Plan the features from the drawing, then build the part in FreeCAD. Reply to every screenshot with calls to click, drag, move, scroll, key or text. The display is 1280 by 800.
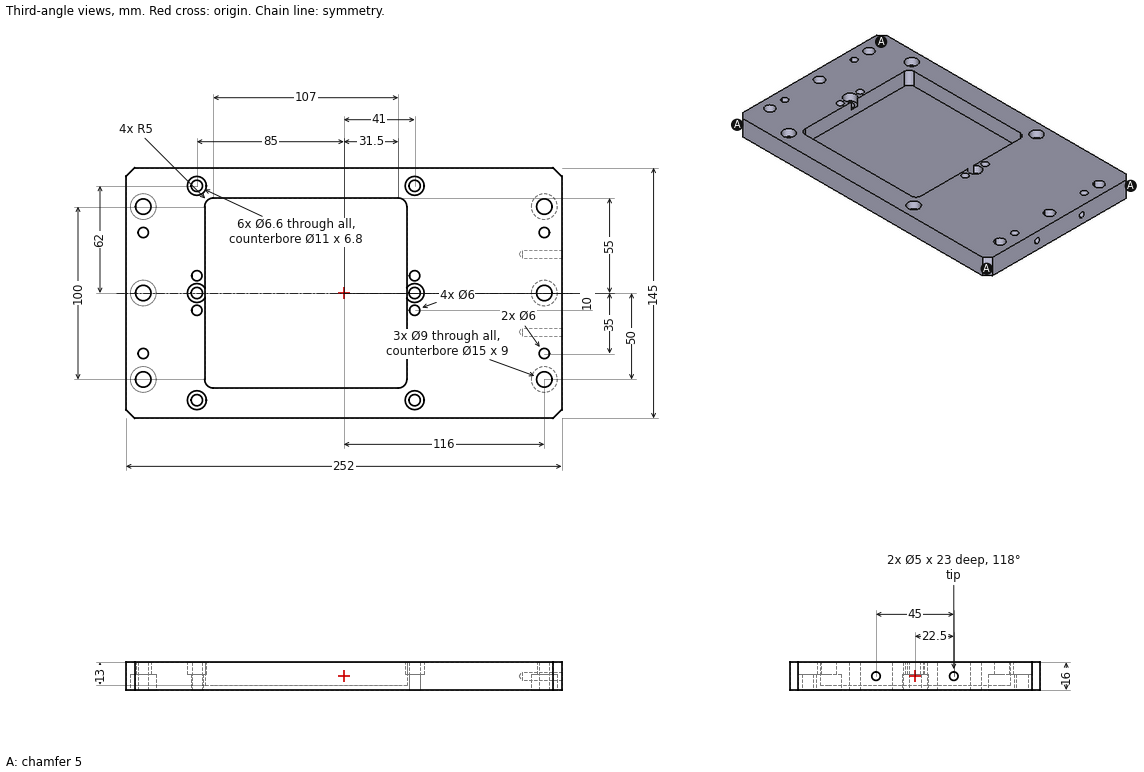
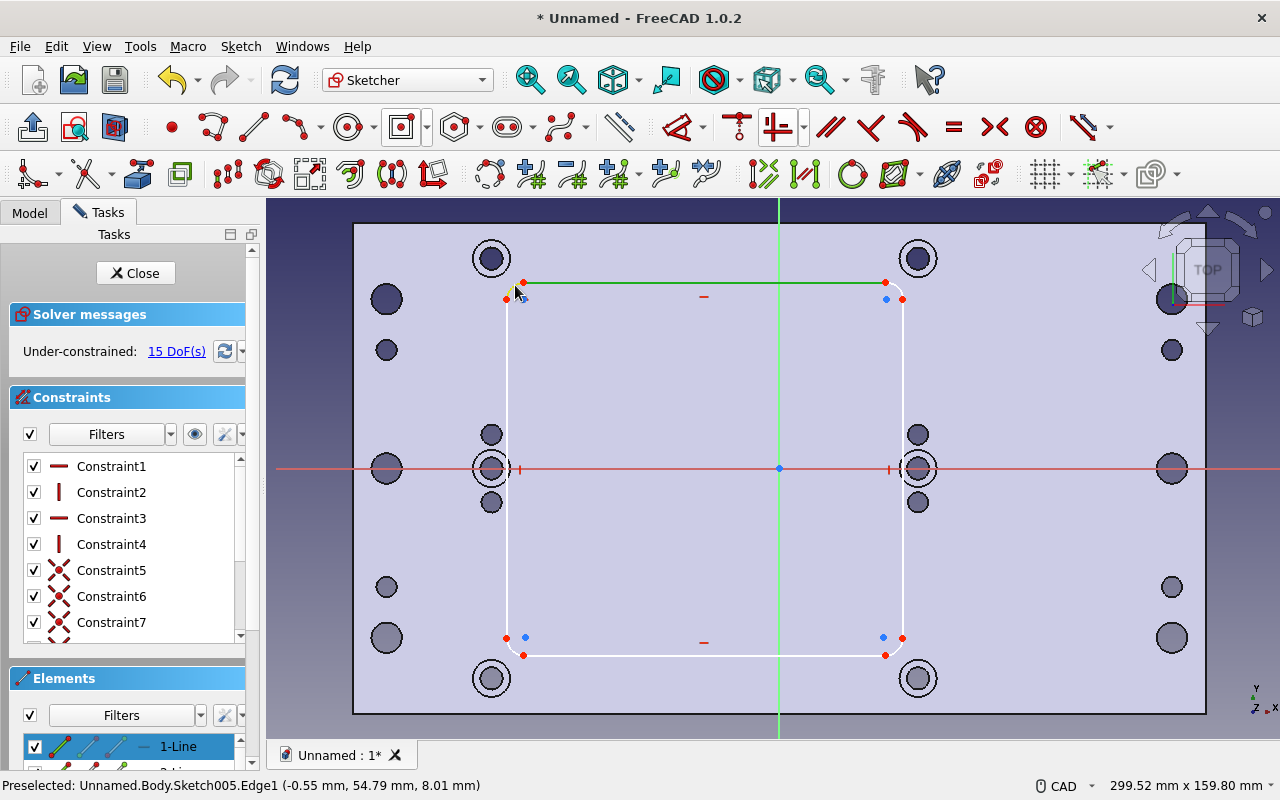
scroll(901, 292, up, 3)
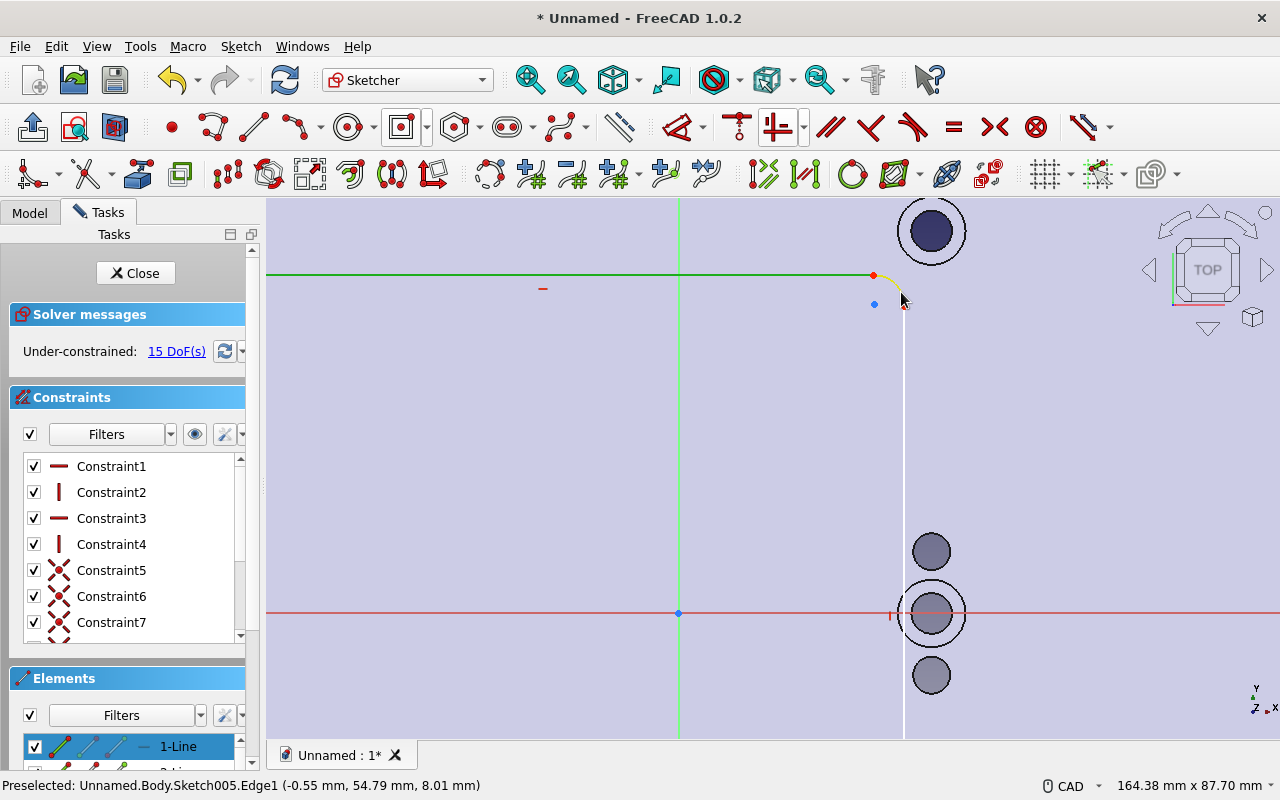
click(901, 292)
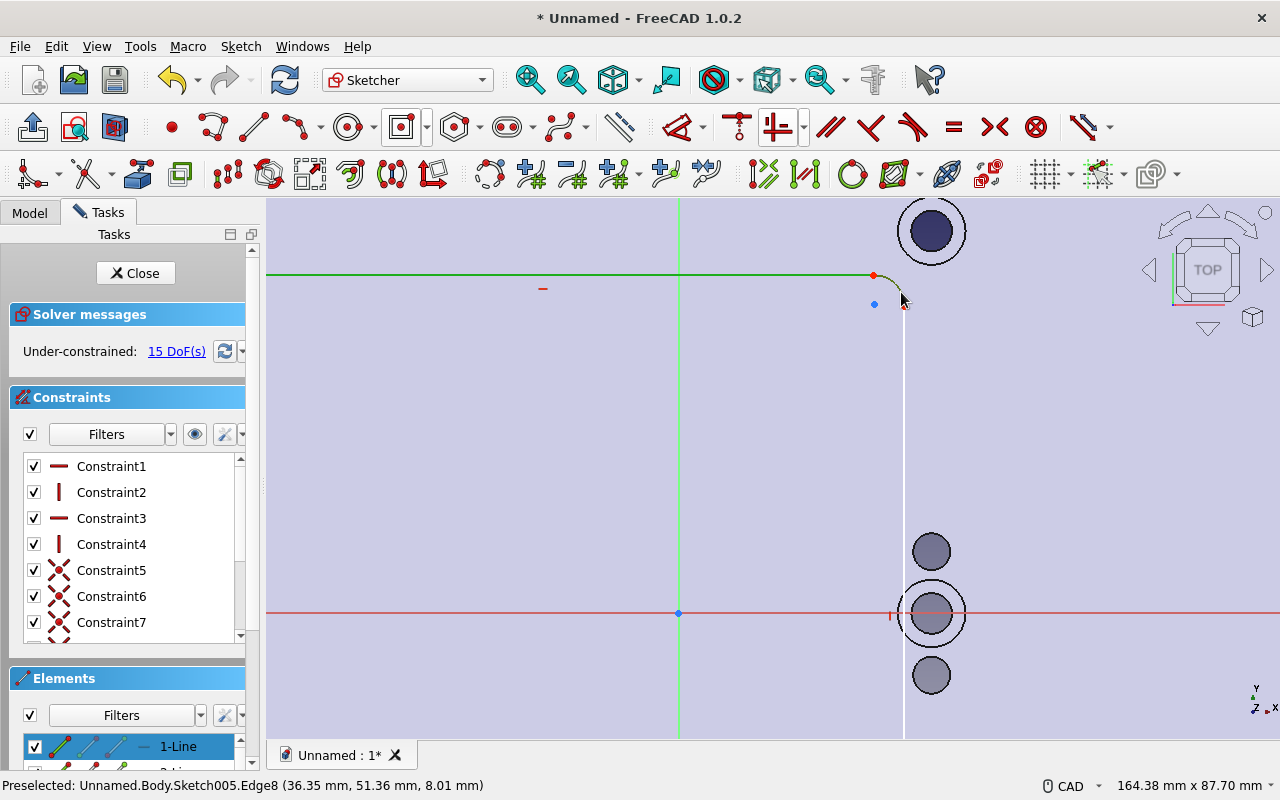
key(t)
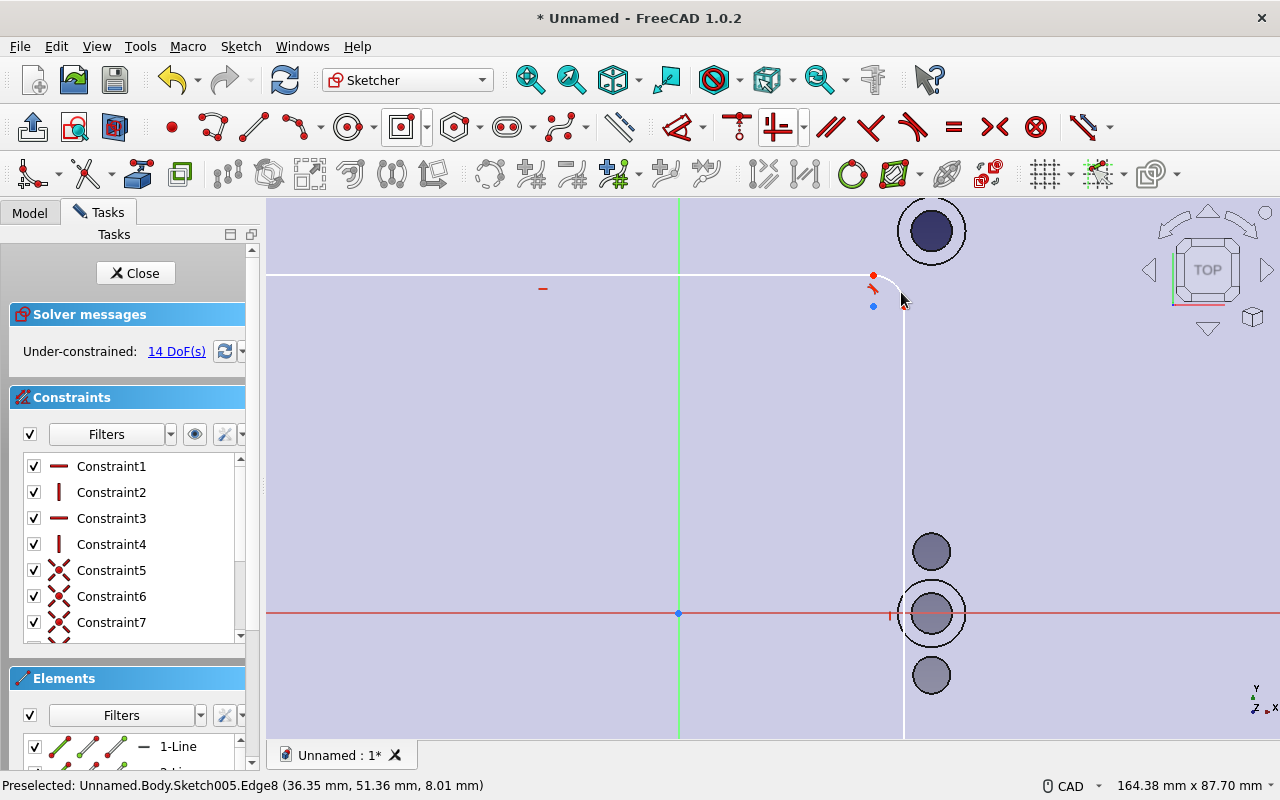
scroll(901, 292, down, 3)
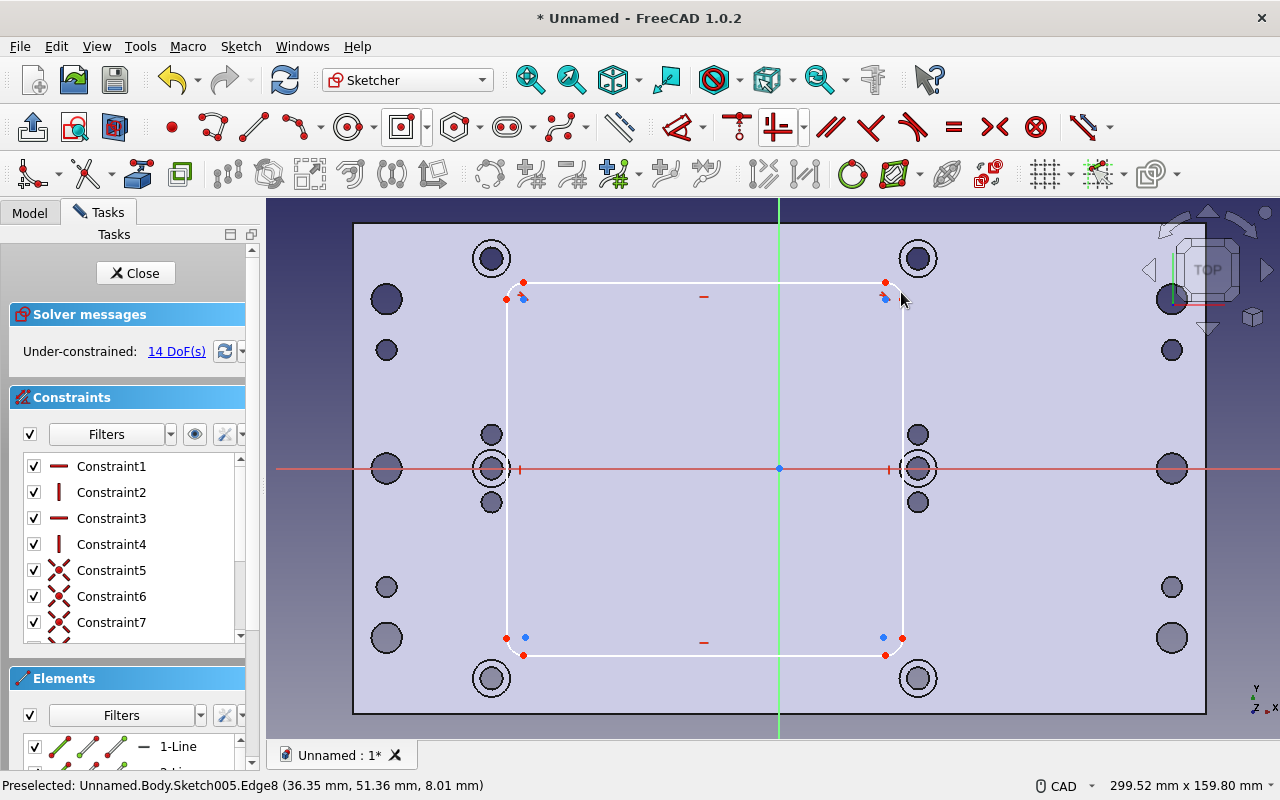
click(507, 402)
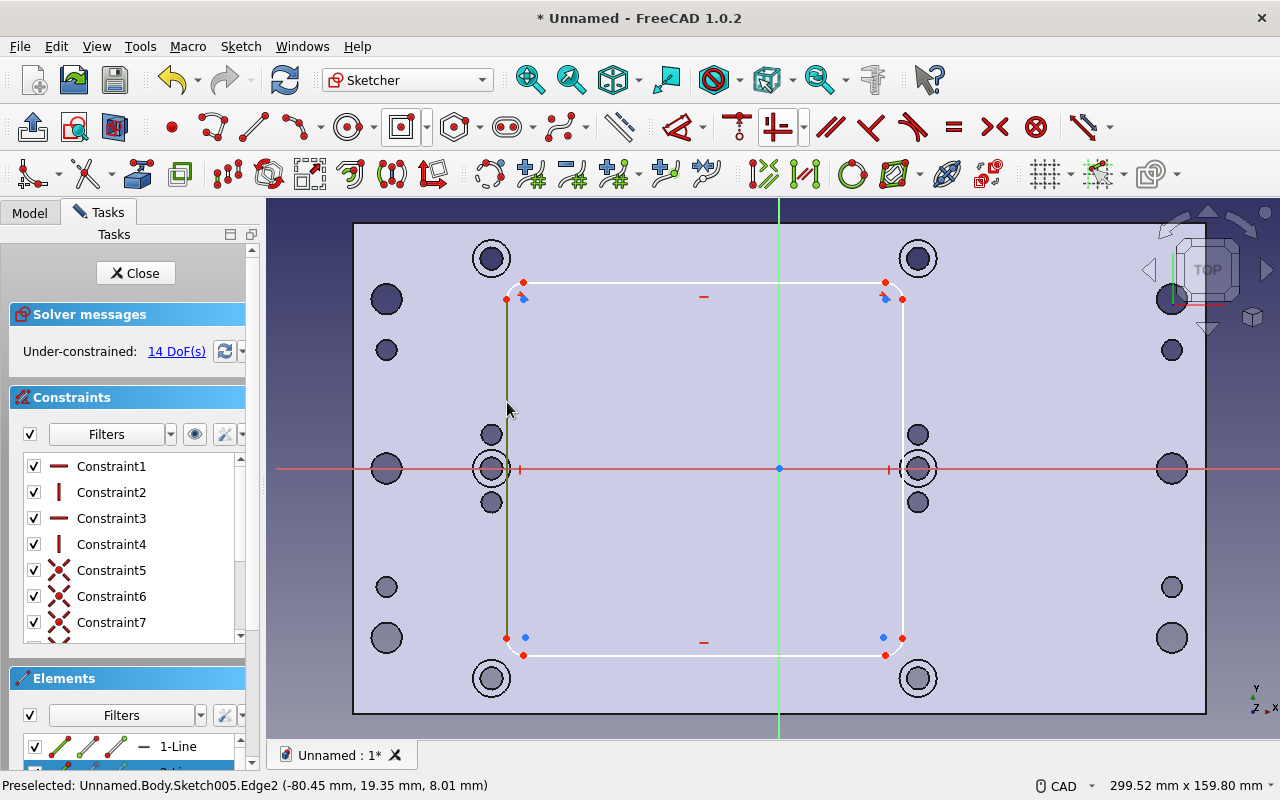
click(512, 288)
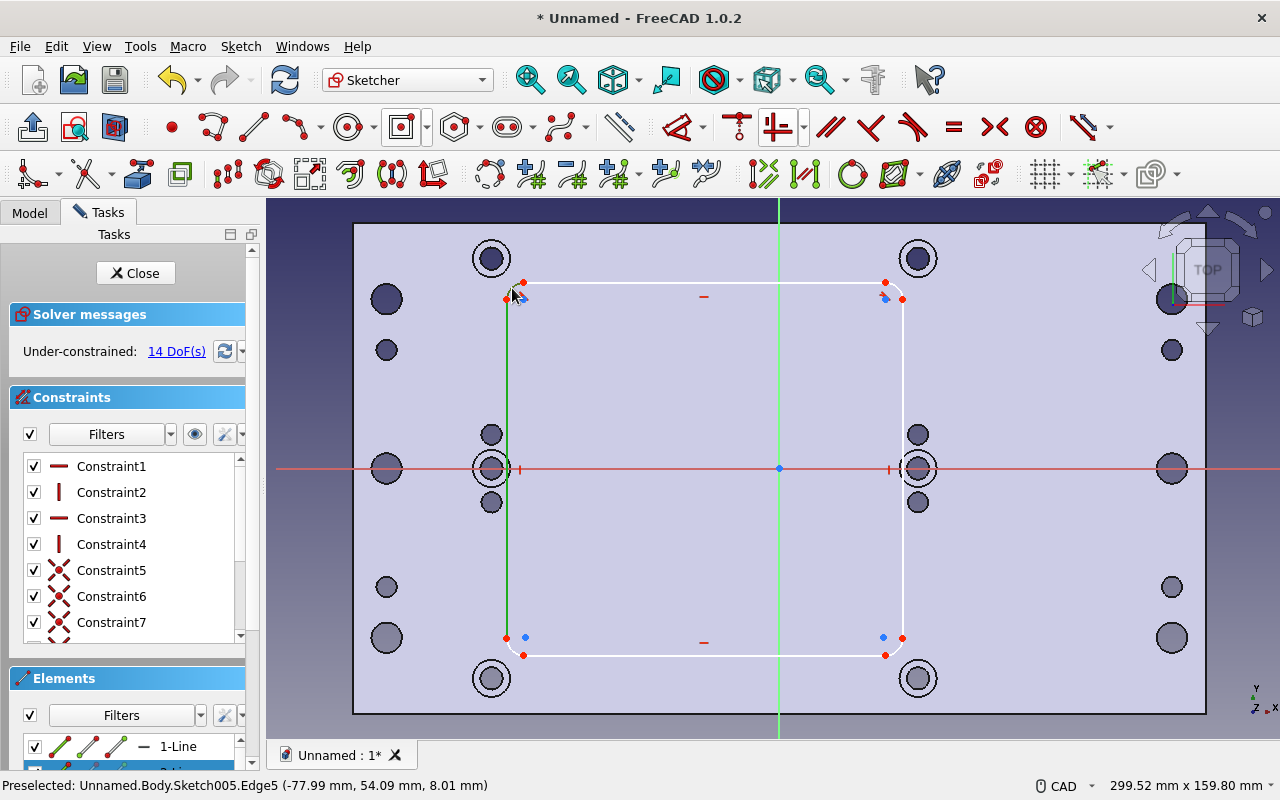
click(913, 128)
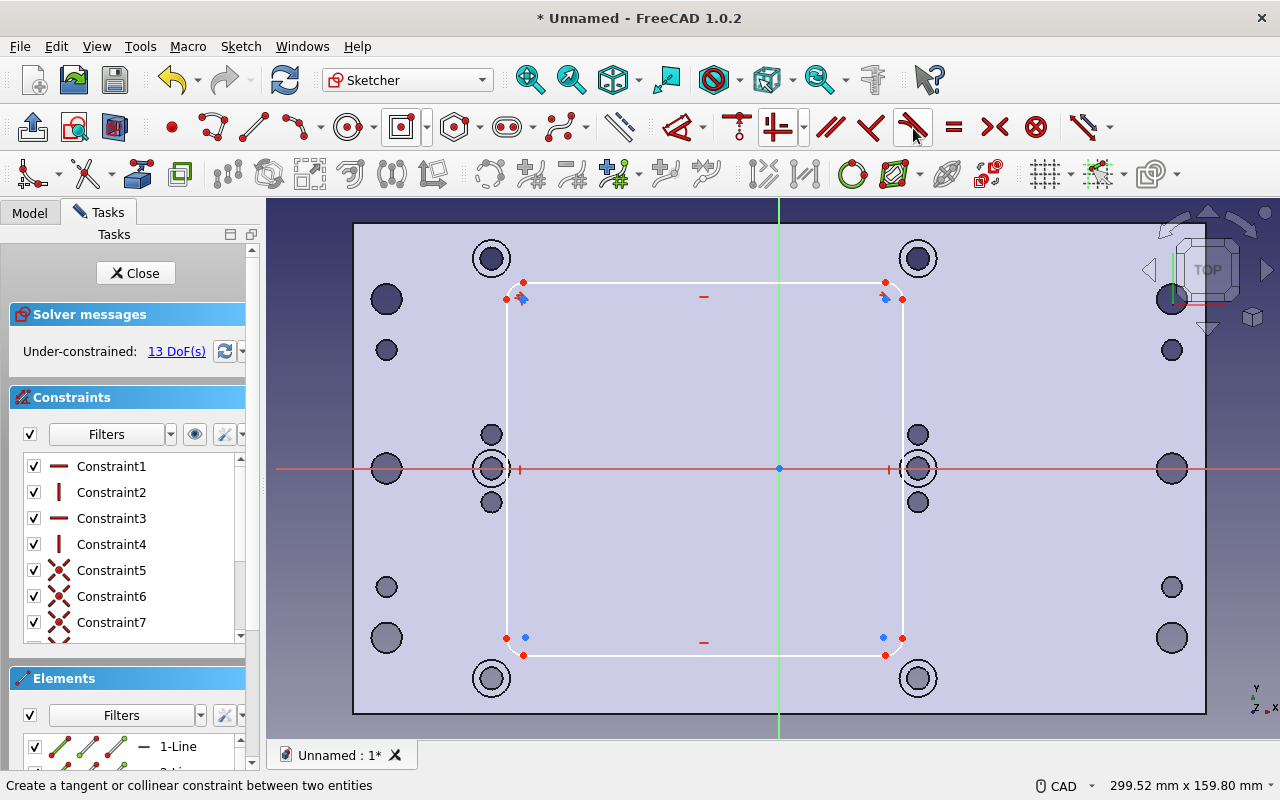
click(507, 402)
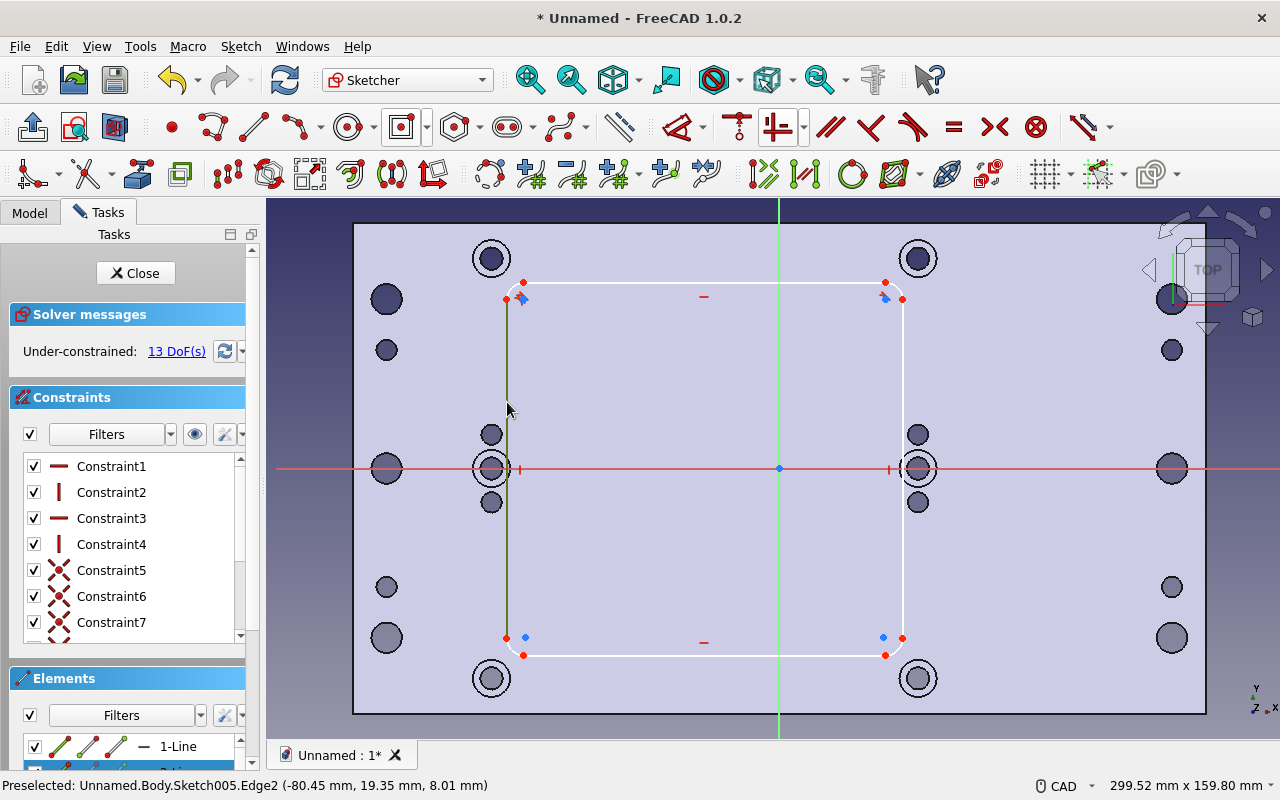
click(512, 651)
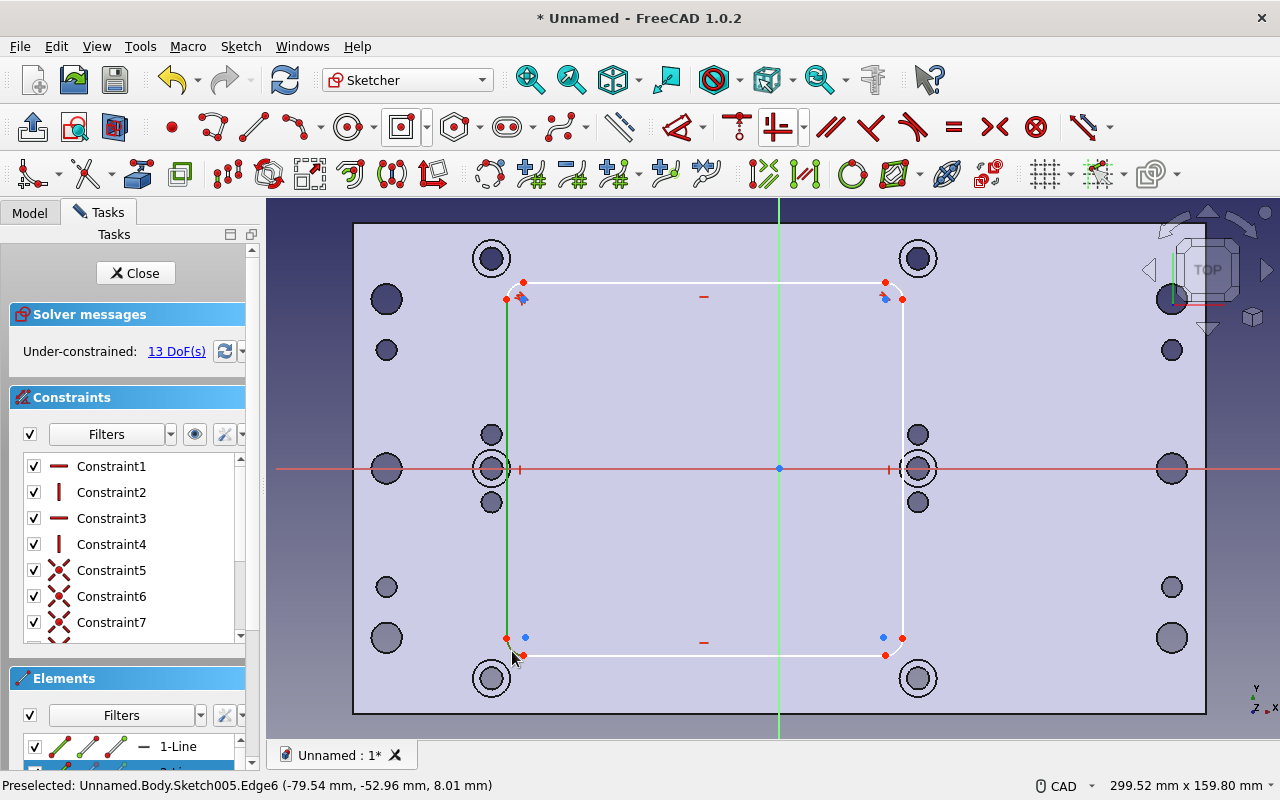
key(t)